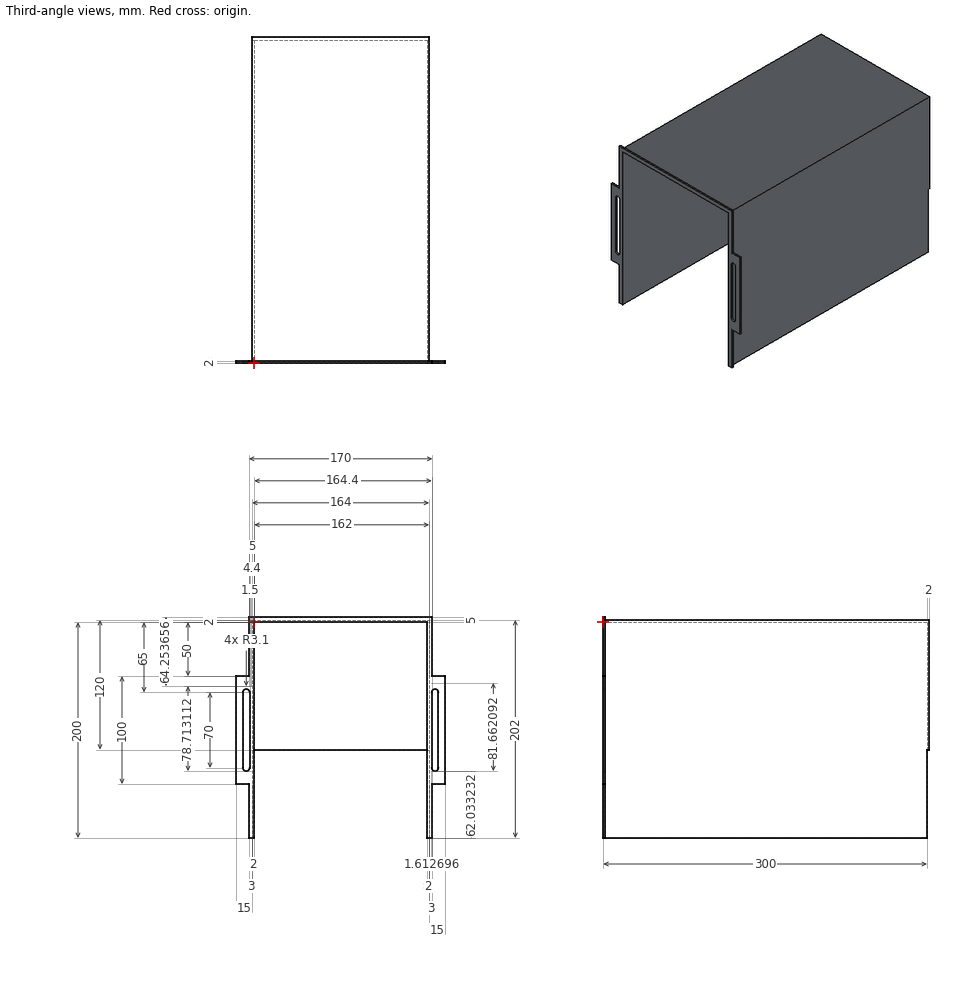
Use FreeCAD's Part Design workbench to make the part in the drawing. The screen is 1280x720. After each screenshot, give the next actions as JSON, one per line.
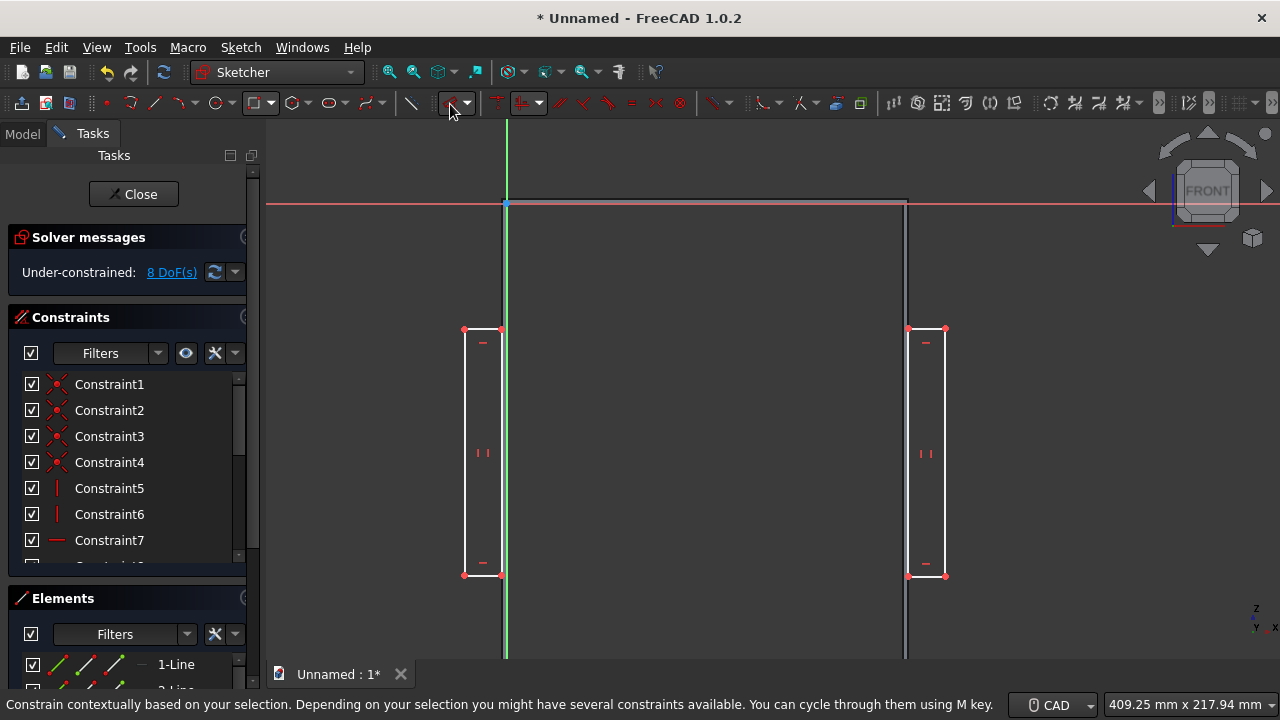
{"action": "scroll", "coordinate": [476, 576], "scroll_direction": "up", "scroll_amount": 2}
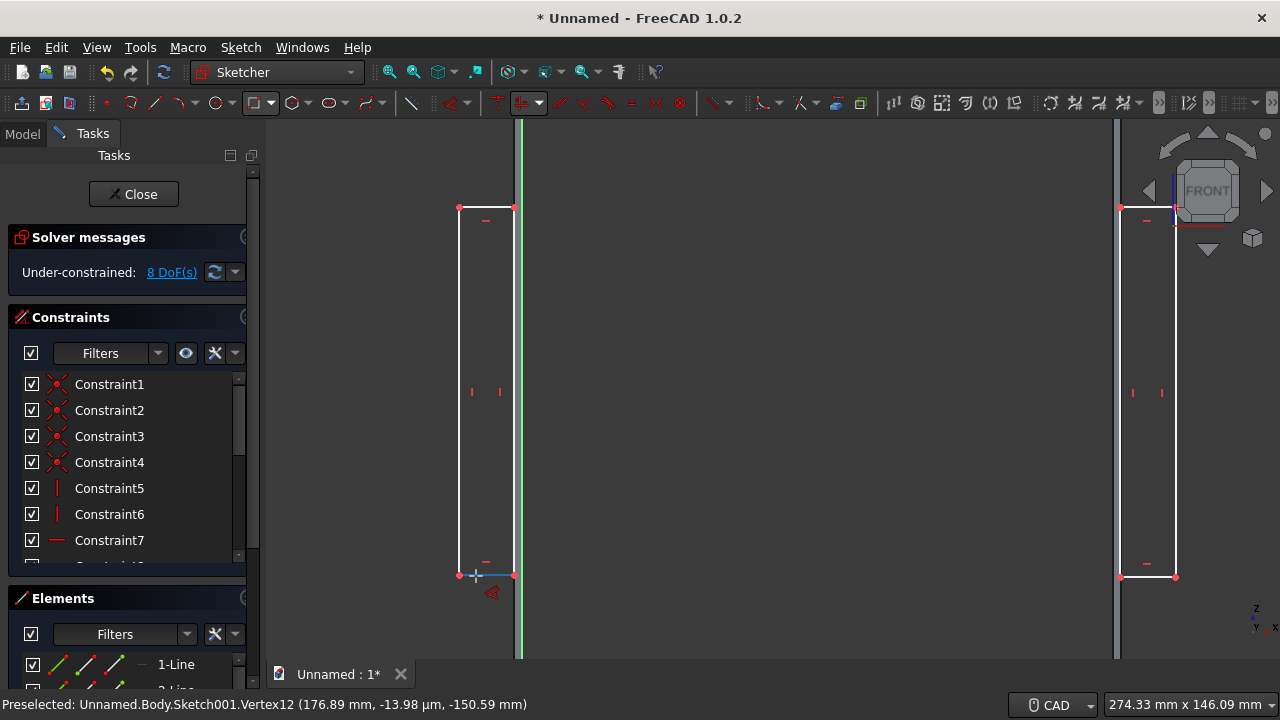
{"action": "left_click", "coordinate": [476, 575]}
{"action": "left_click", "coordinate": [487, 609]}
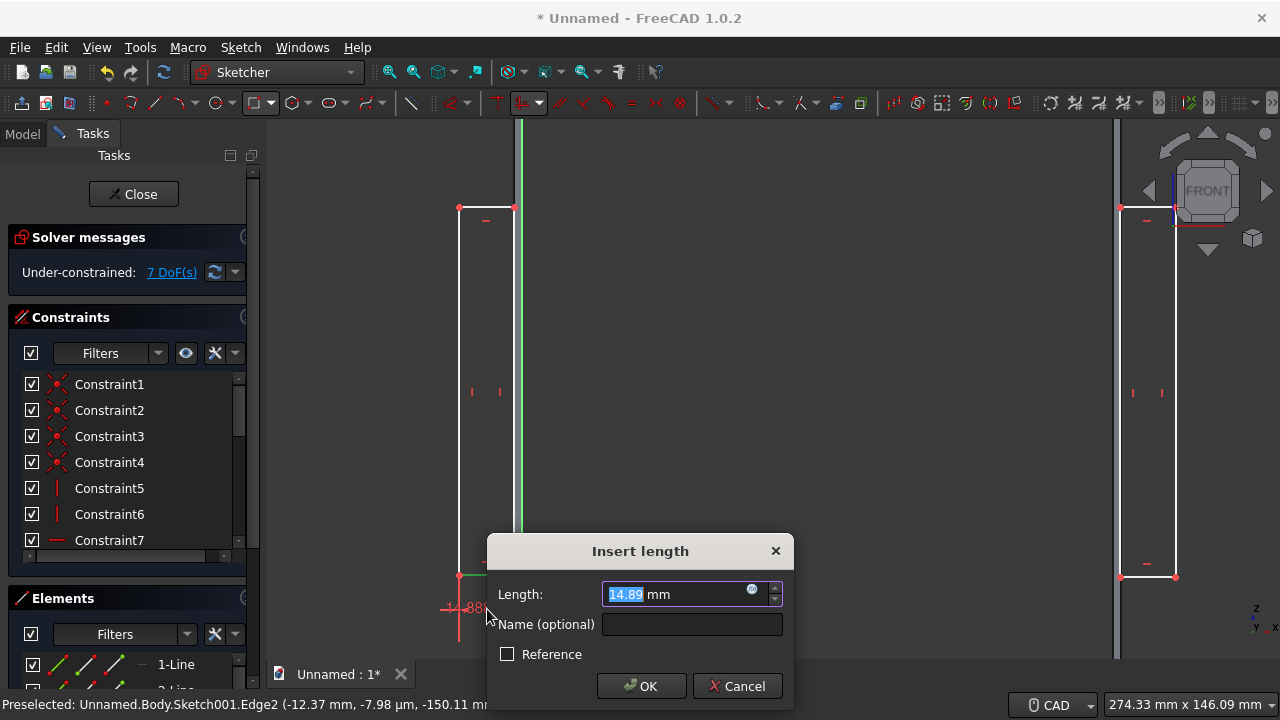
{"action": "type", "text": "15"}
{"action": "key", "text": "Return"}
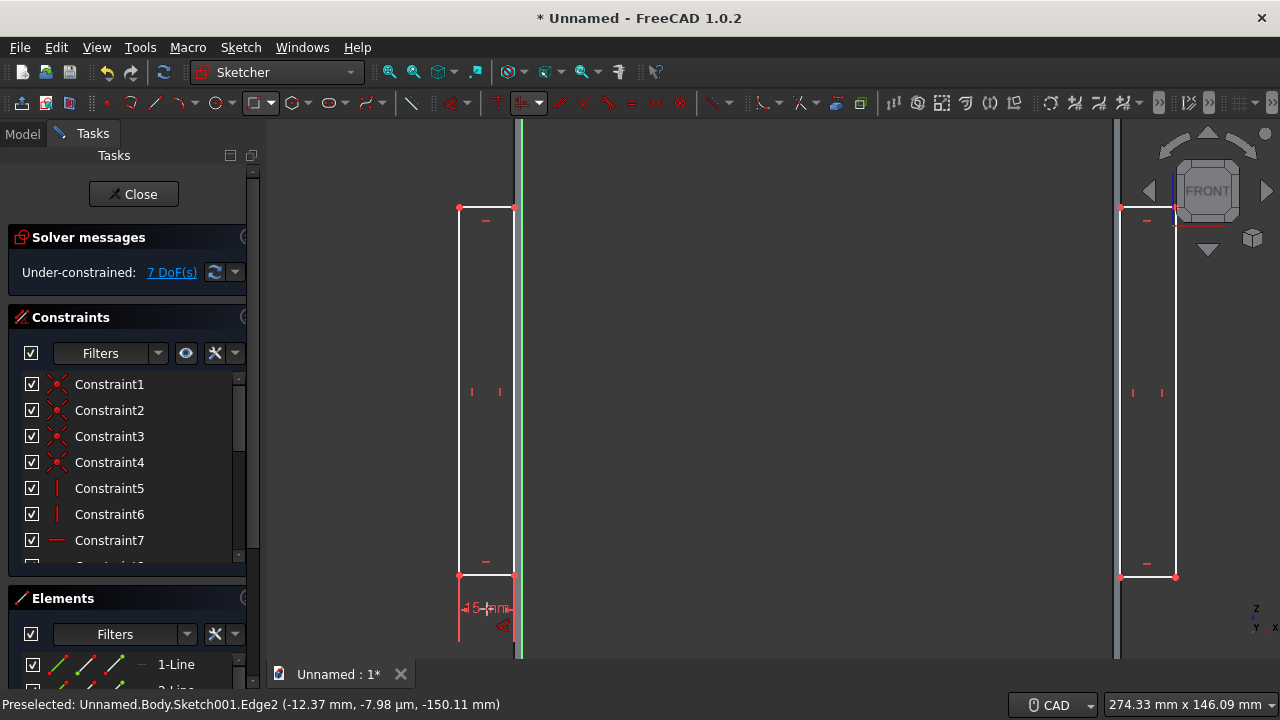
{"action": "scroll", "coordinate": [475, 575], "scroll_direction": "down", "scroll_amount": 2}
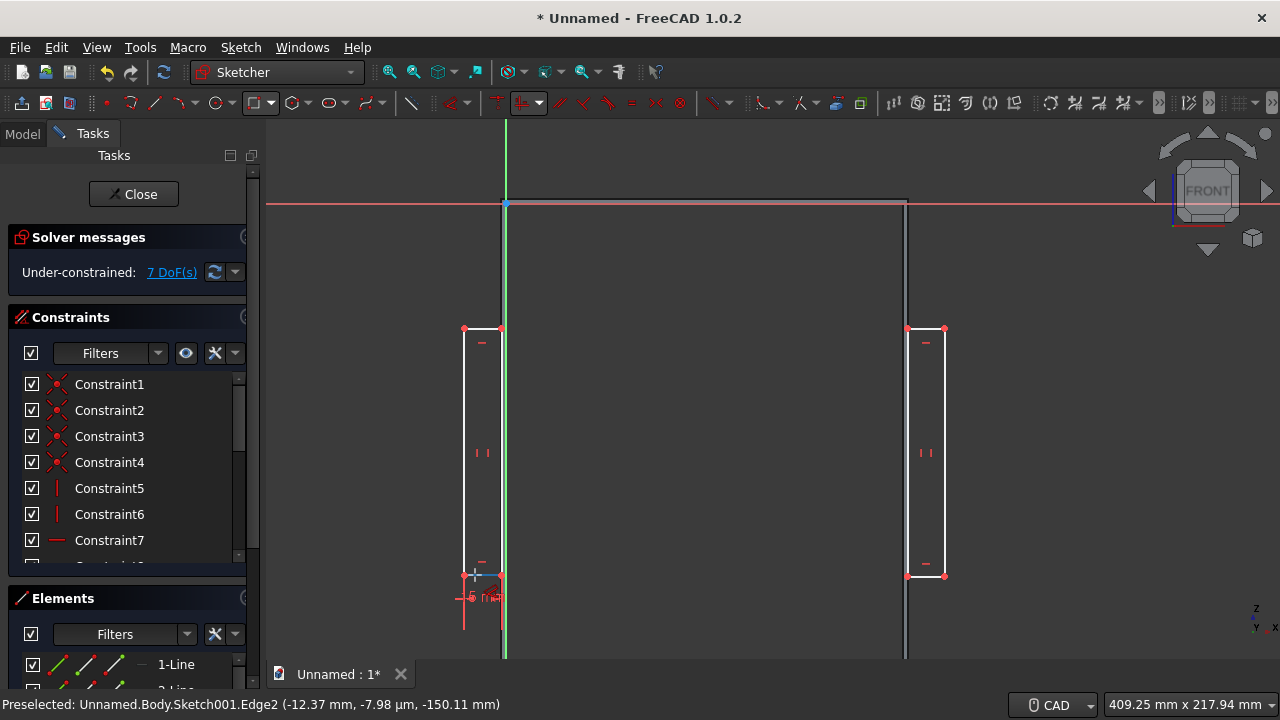
{"action": "scroll", "coordinate": [919, 577], "scroll_direction": "up", "scroll_amount": 2}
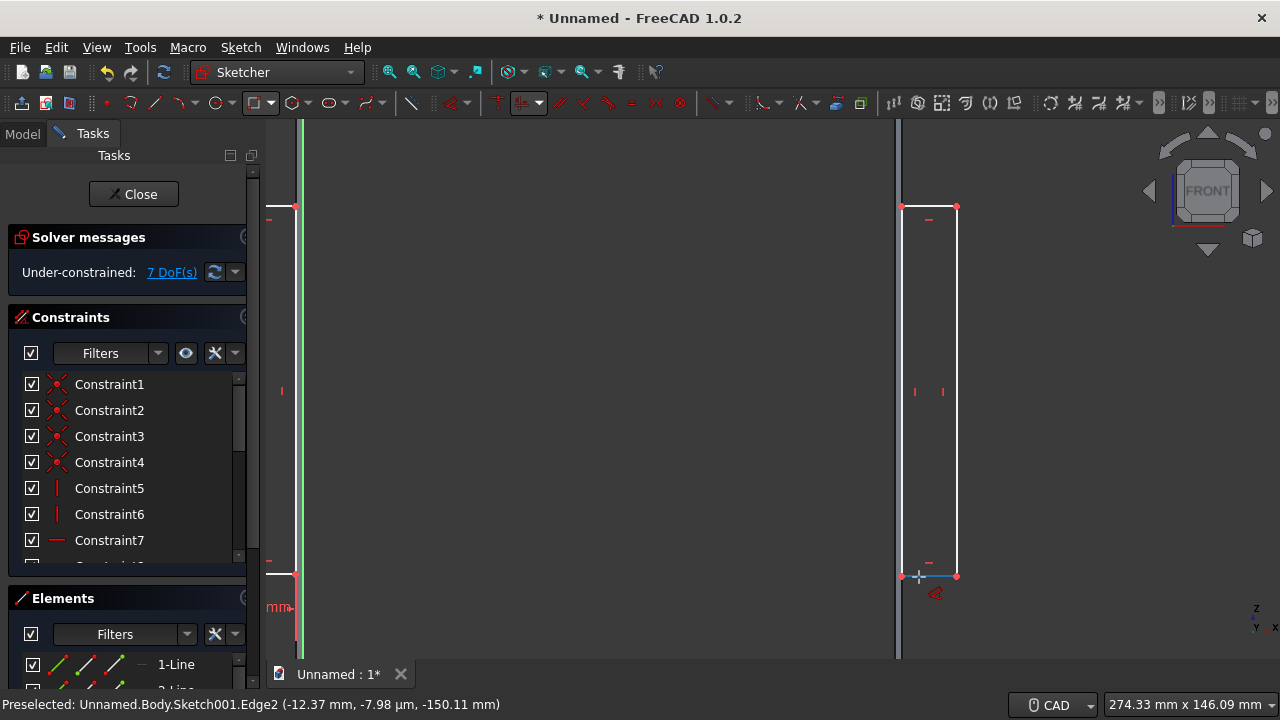
{"action": "left_click", "coordinate": [918, 576]}
{"action": "left_click", "coordinate": [929, 610]}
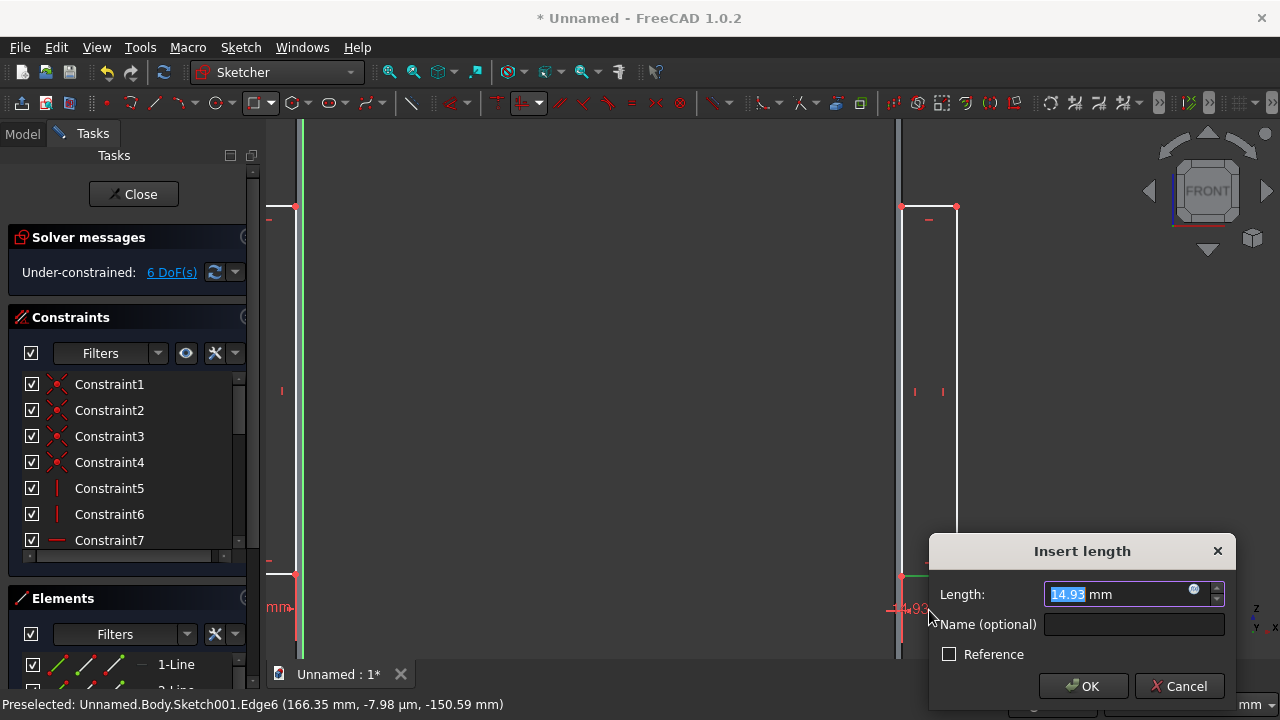
{"action": "type", "text": "15"}
{"action": "key", "text": "Return"}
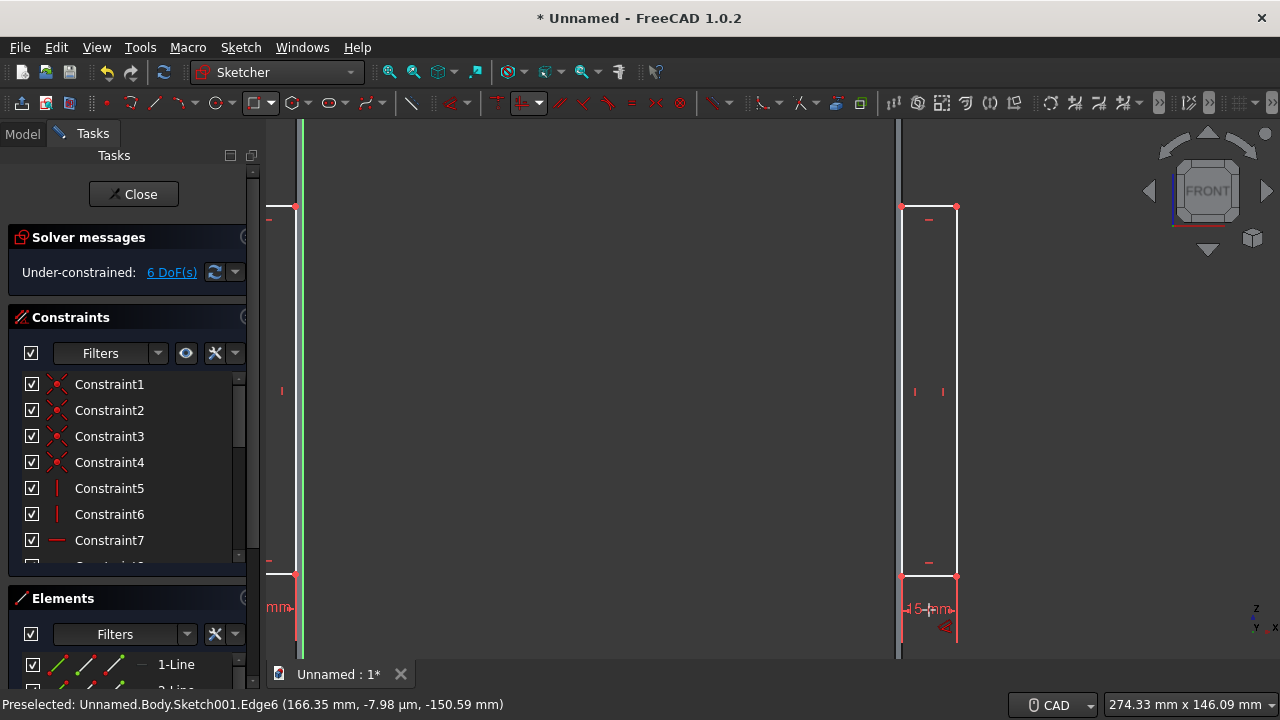
{"action": "scroll", "coordinate": [296, 574], "scroll_direction": "up", "scroll_amount": 9}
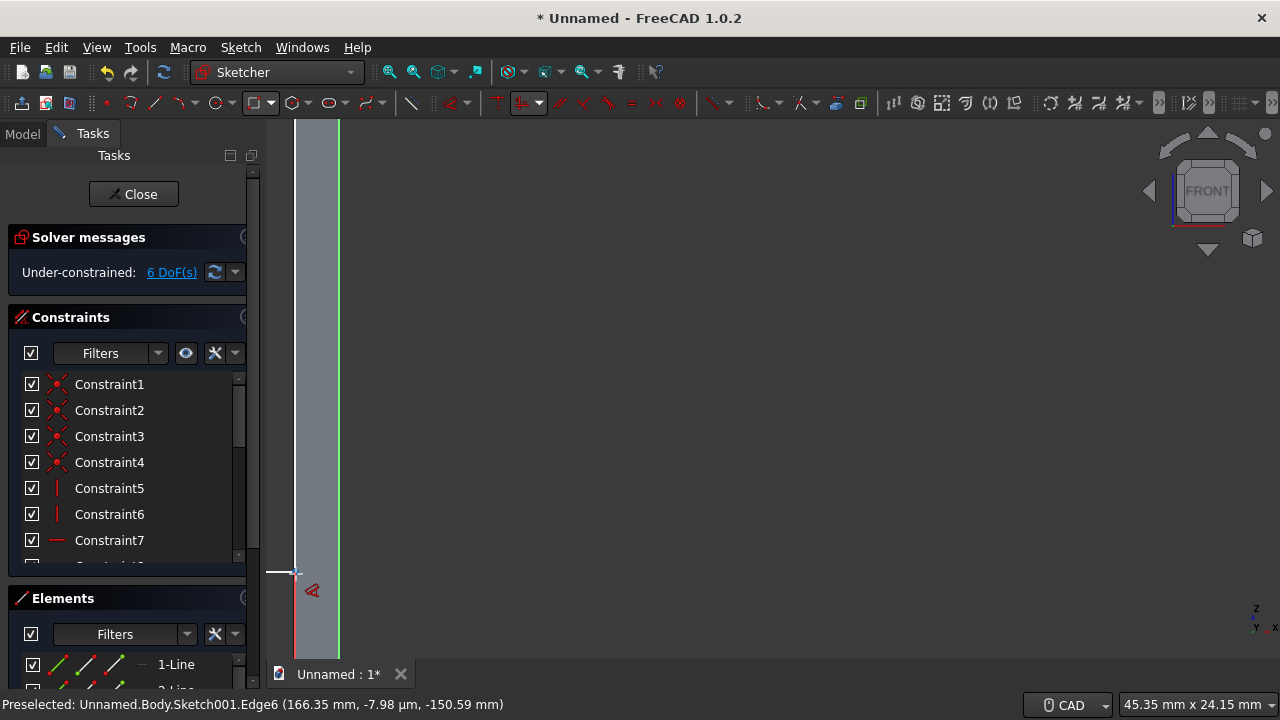
{"action": "left_click", "coordinate": [295, 572]}
{"action": "left_click", "coordinate": [317, 606]}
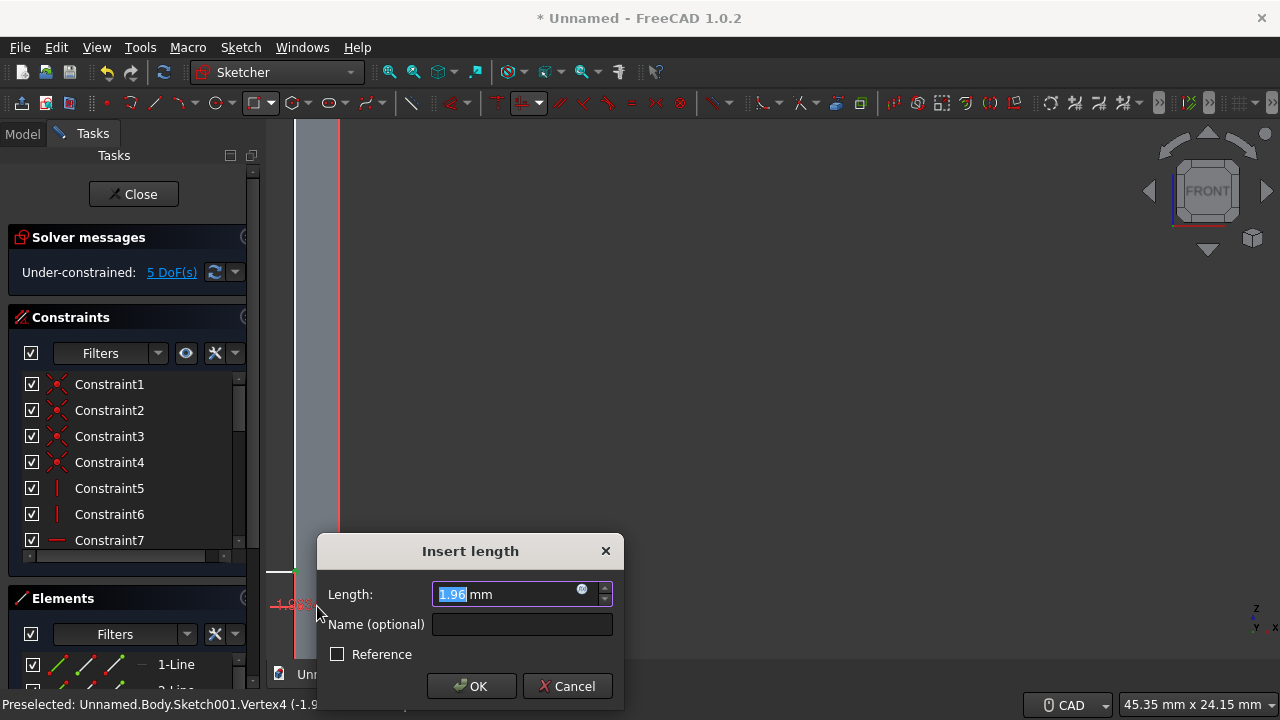
{"action": "type", "text": "2"}
{"action": "key", "text": "Return"}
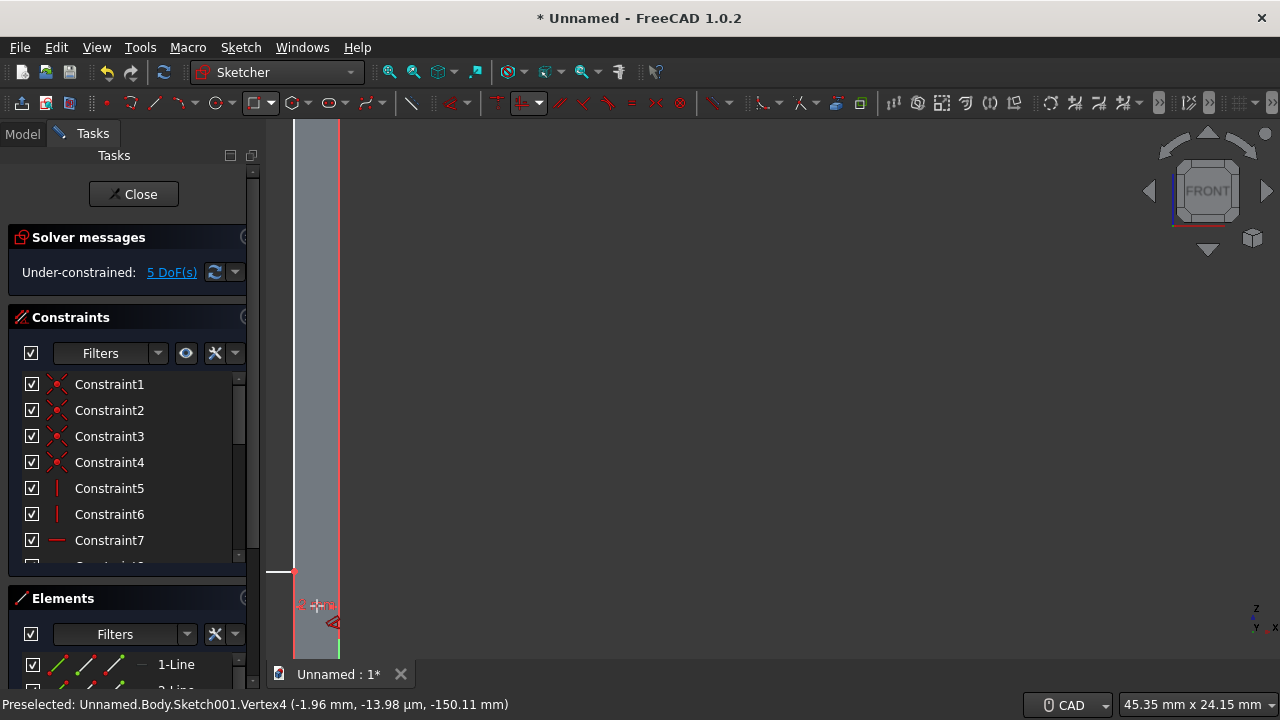
{"action": "scroll", "coordinate": [527, 576], "scroll_direction": "down", "scroll_amount": 11}